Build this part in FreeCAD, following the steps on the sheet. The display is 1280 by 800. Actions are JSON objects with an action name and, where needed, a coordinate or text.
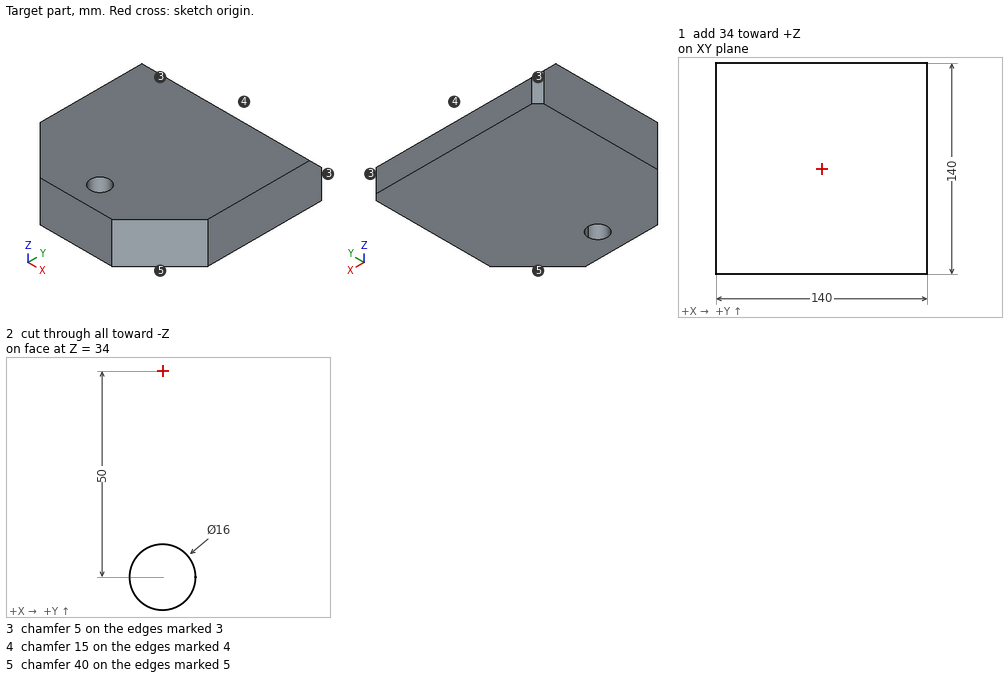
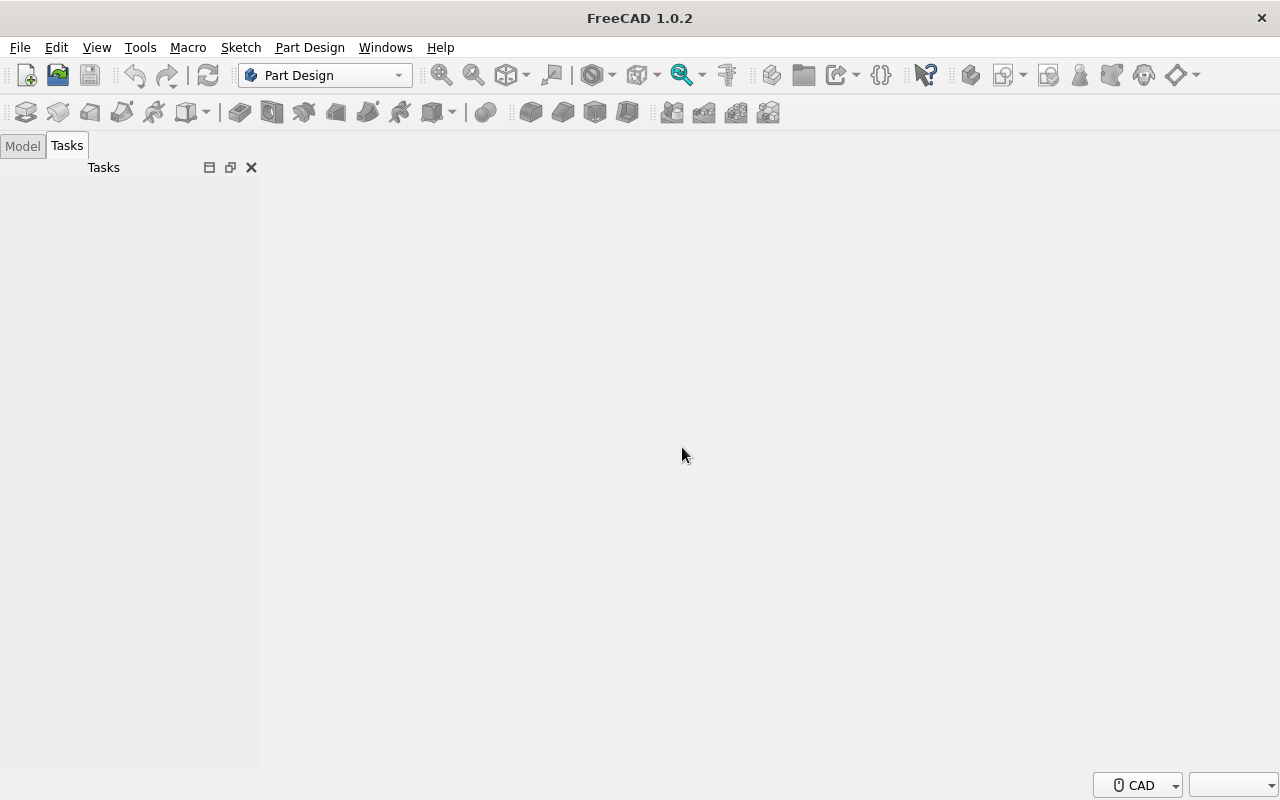
{"action": "key", "text": "ctrl+n"}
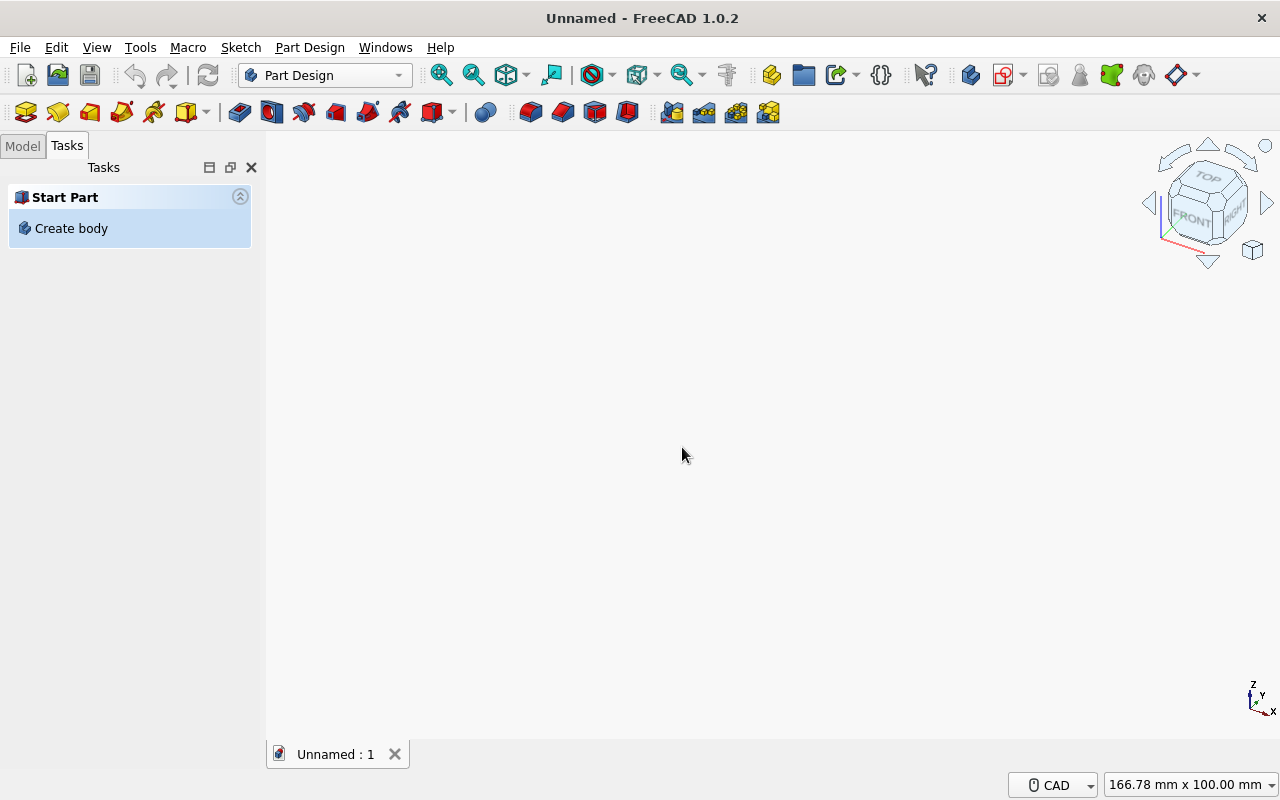
{"action": "left_click", "coordinate": [1004, 76]}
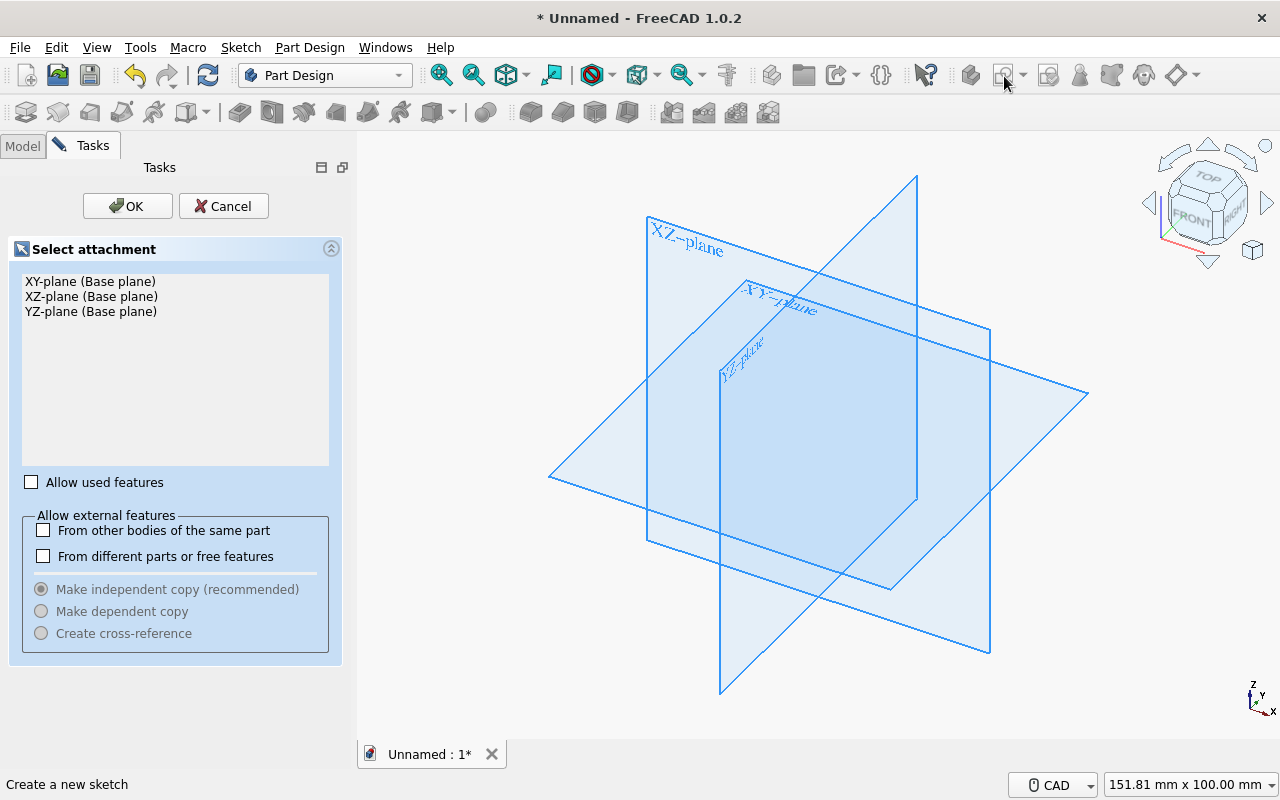
{"action": "left_click", "coordinate": [82, 282]}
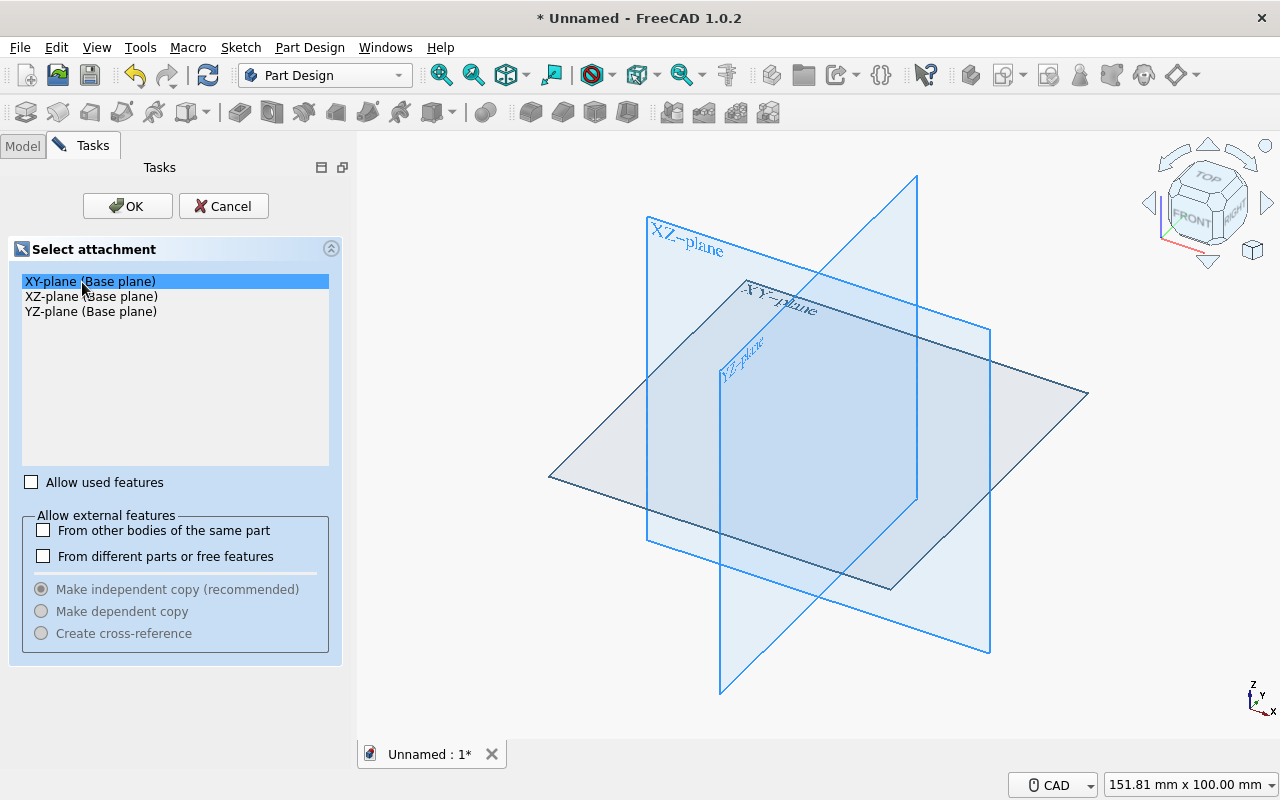
{"action": "left_click", "coordinate": [128, 206]}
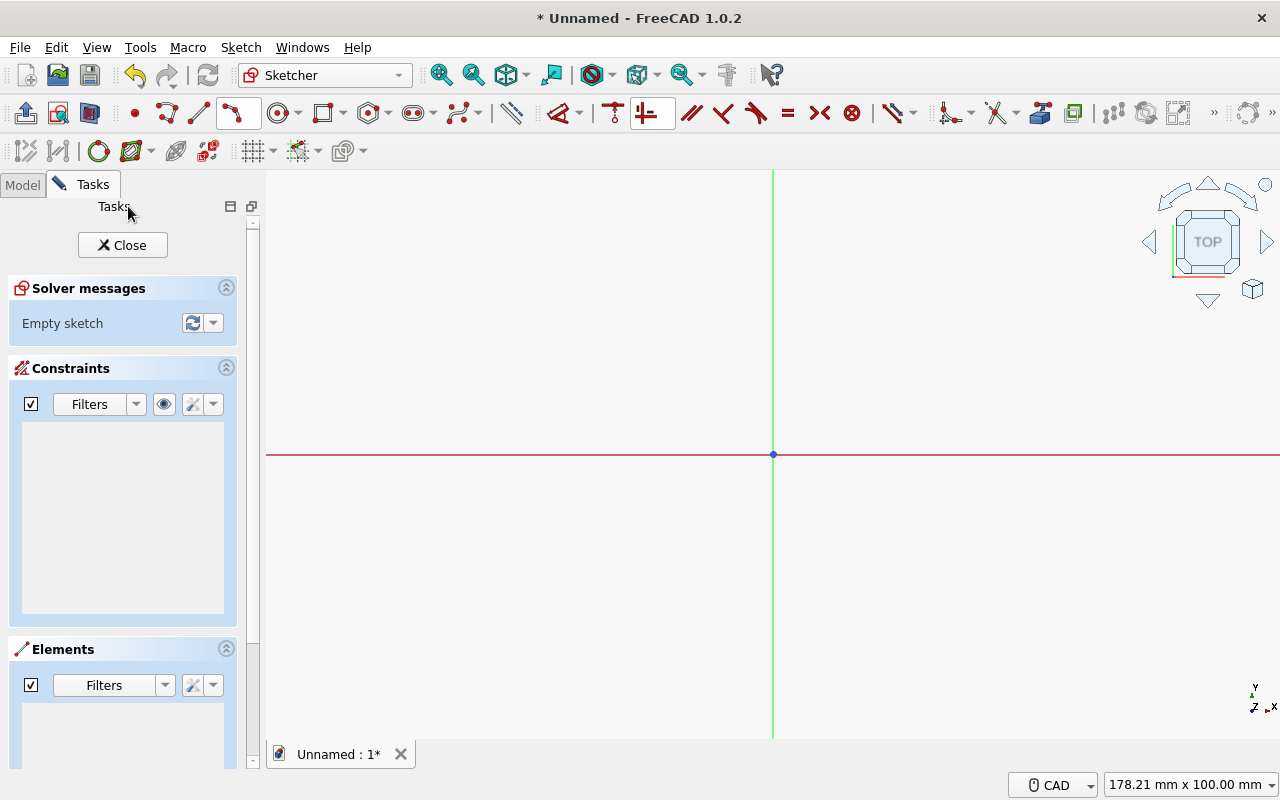
{"action": "scroll", "coordinate": [649, 454], "scroll_direction": "down", "scroll_amount": 4}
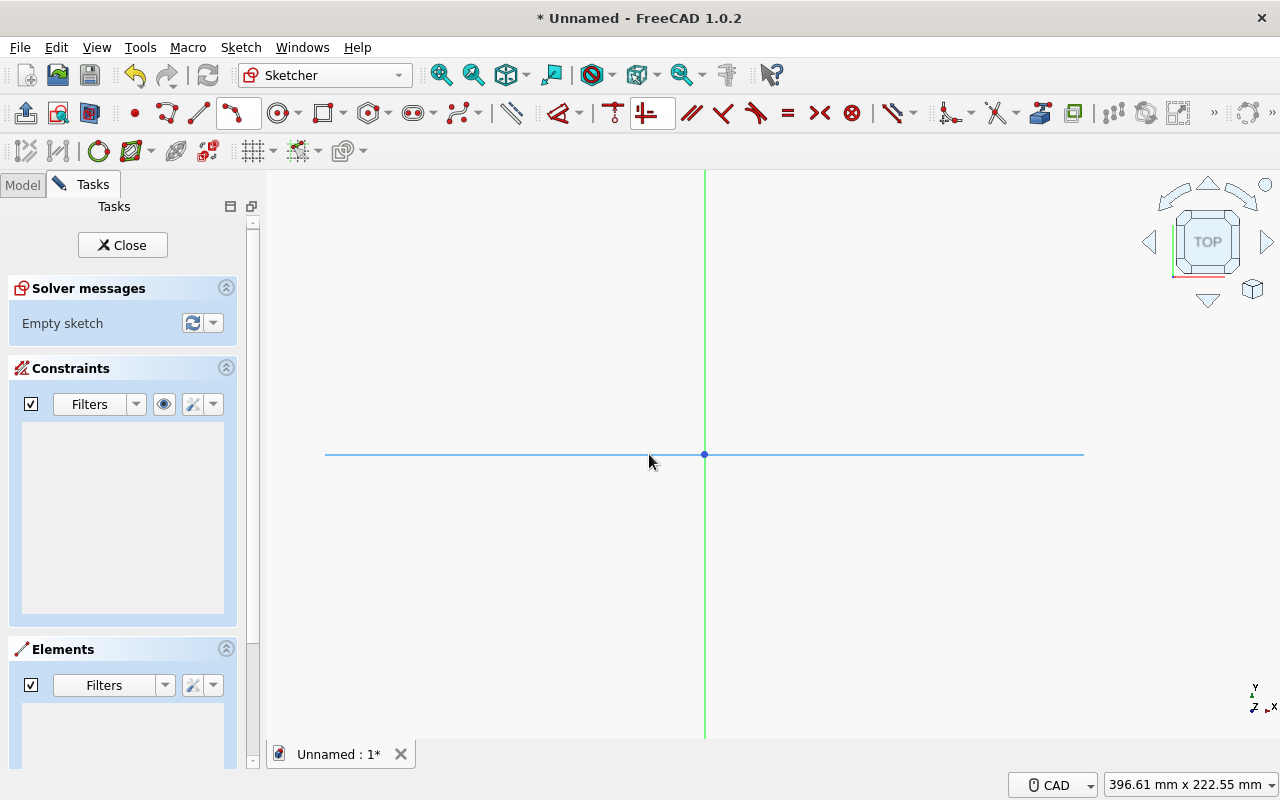
{"action": "key", "text": "g v"}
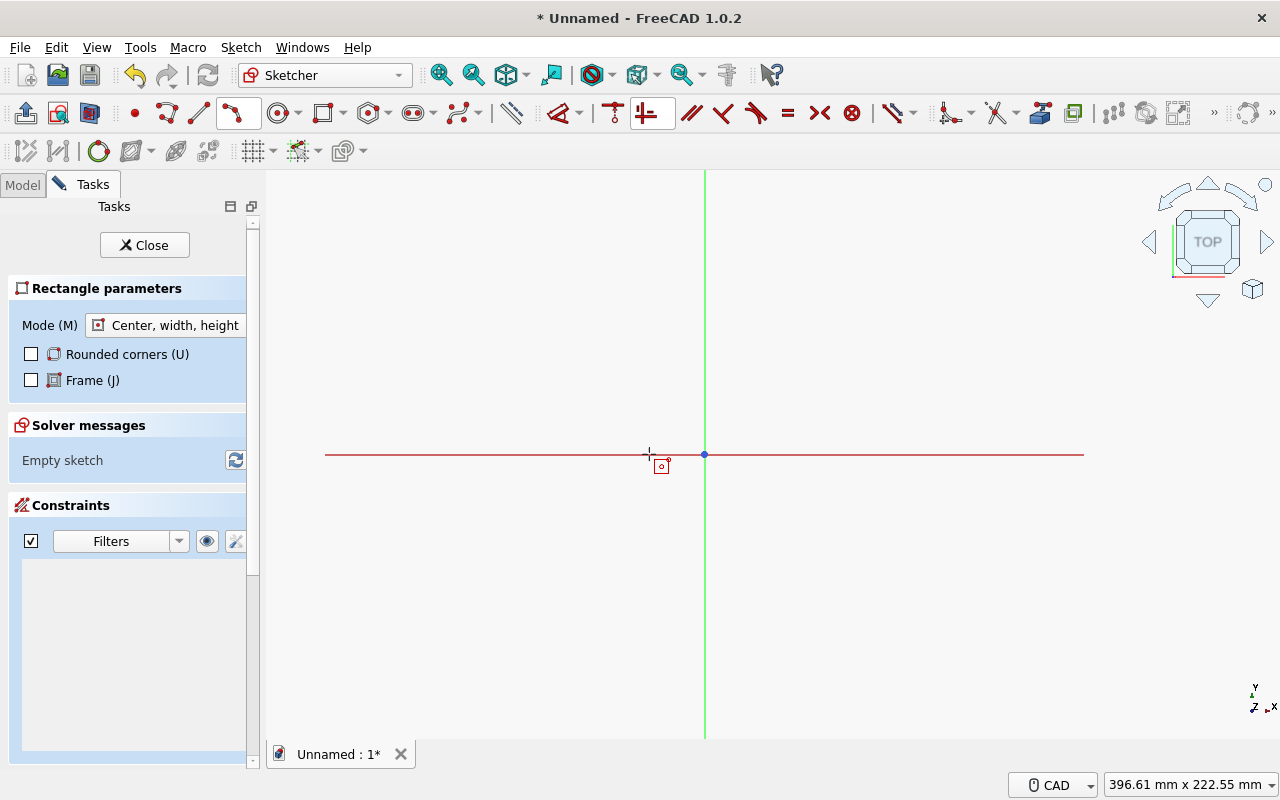
{"action": "left_click", "coordinate": [705, 454]}
{"action": "left_click", "coordinate": [884, 276]}
{"action": "key", "text": "Escape"}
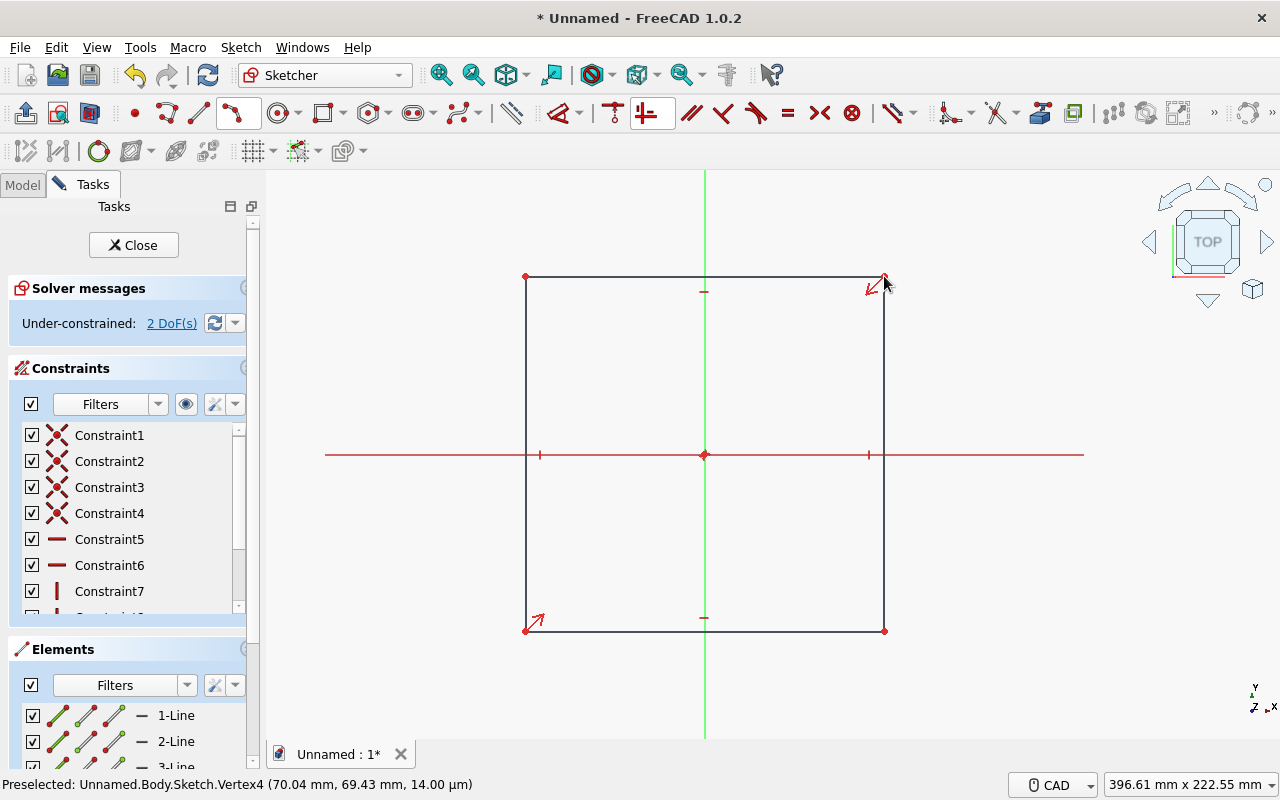
{"action": "key", "text": "d"}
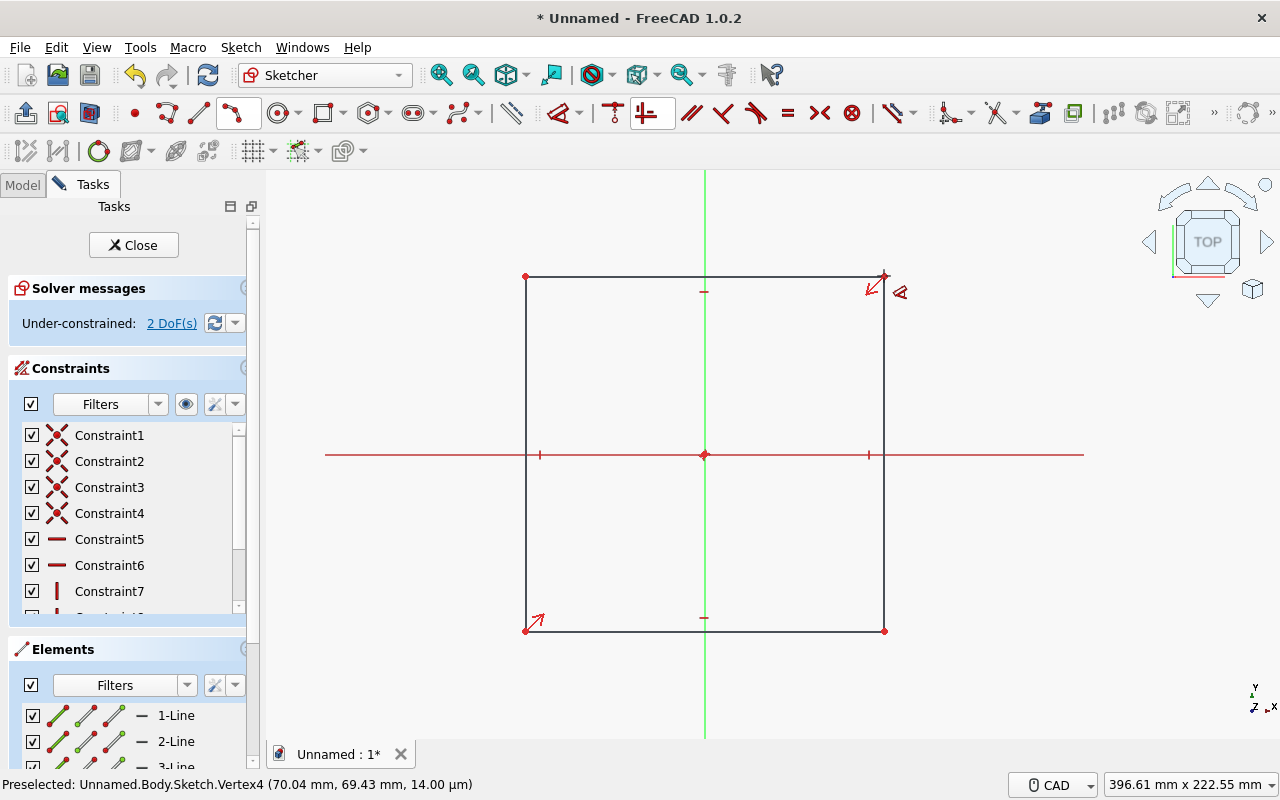
{"action": "left_click", "coordinate": [633, 632]}
{"action": "left_click", "coordinate": [623, 666]}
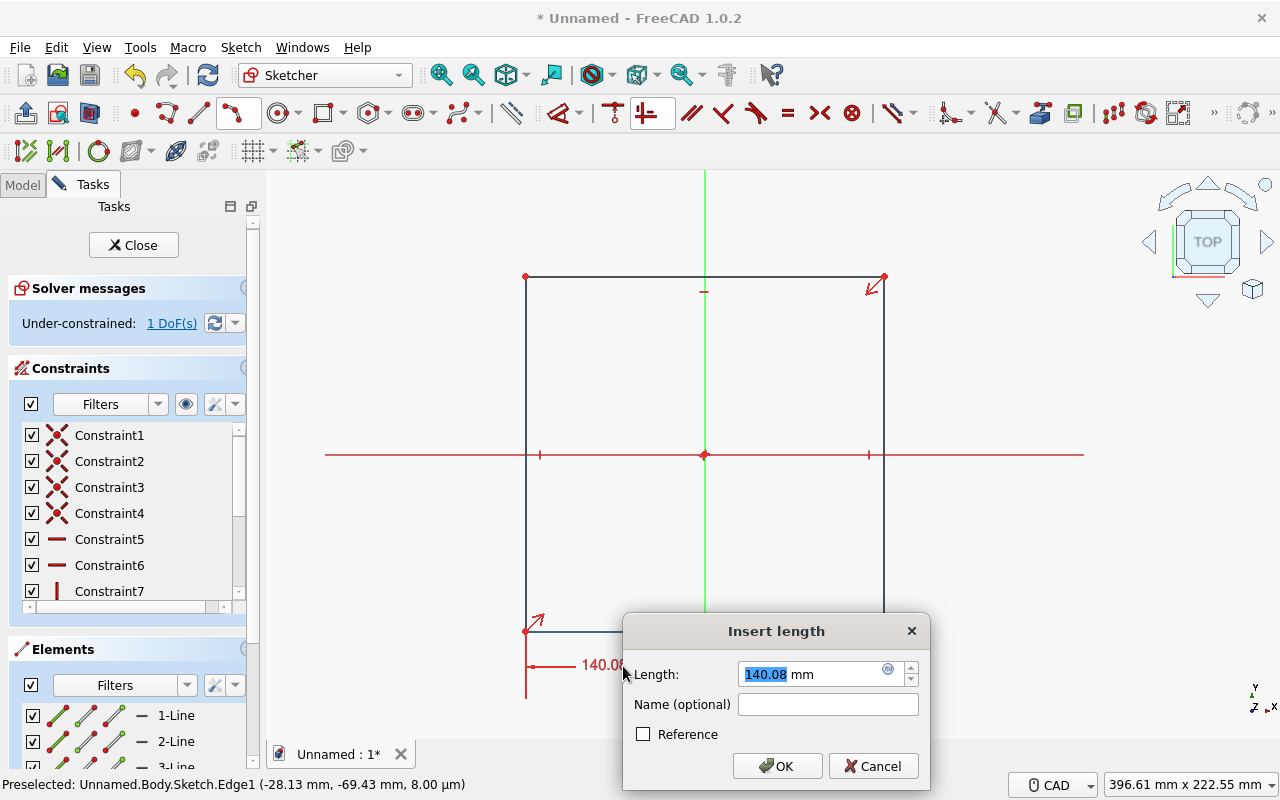
{"action": "type", "text": "140"}
{"action": "key", "text": "Return"}